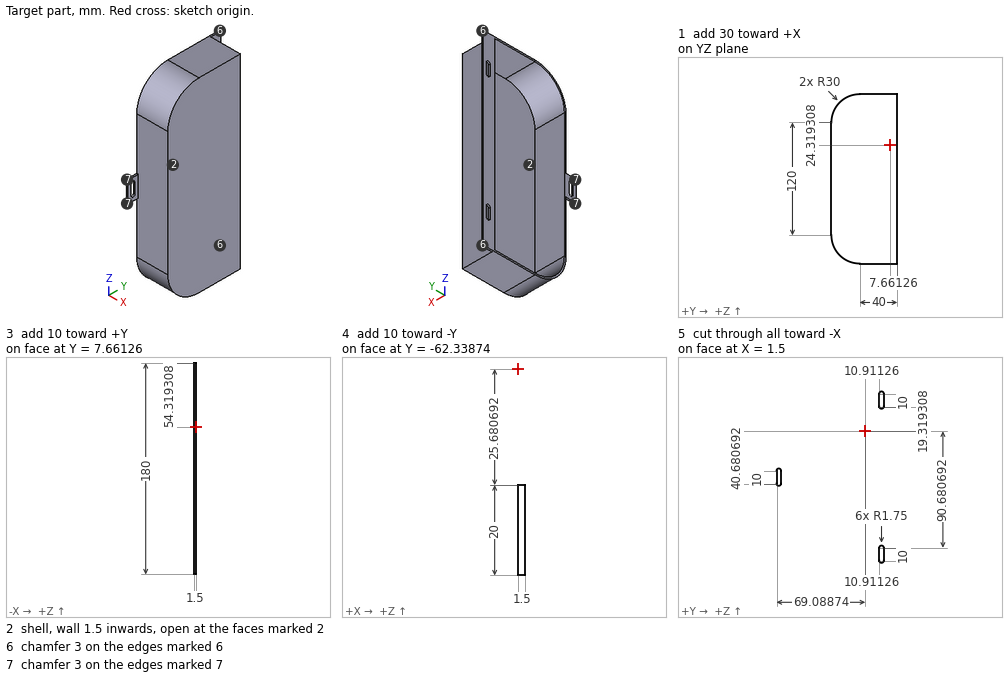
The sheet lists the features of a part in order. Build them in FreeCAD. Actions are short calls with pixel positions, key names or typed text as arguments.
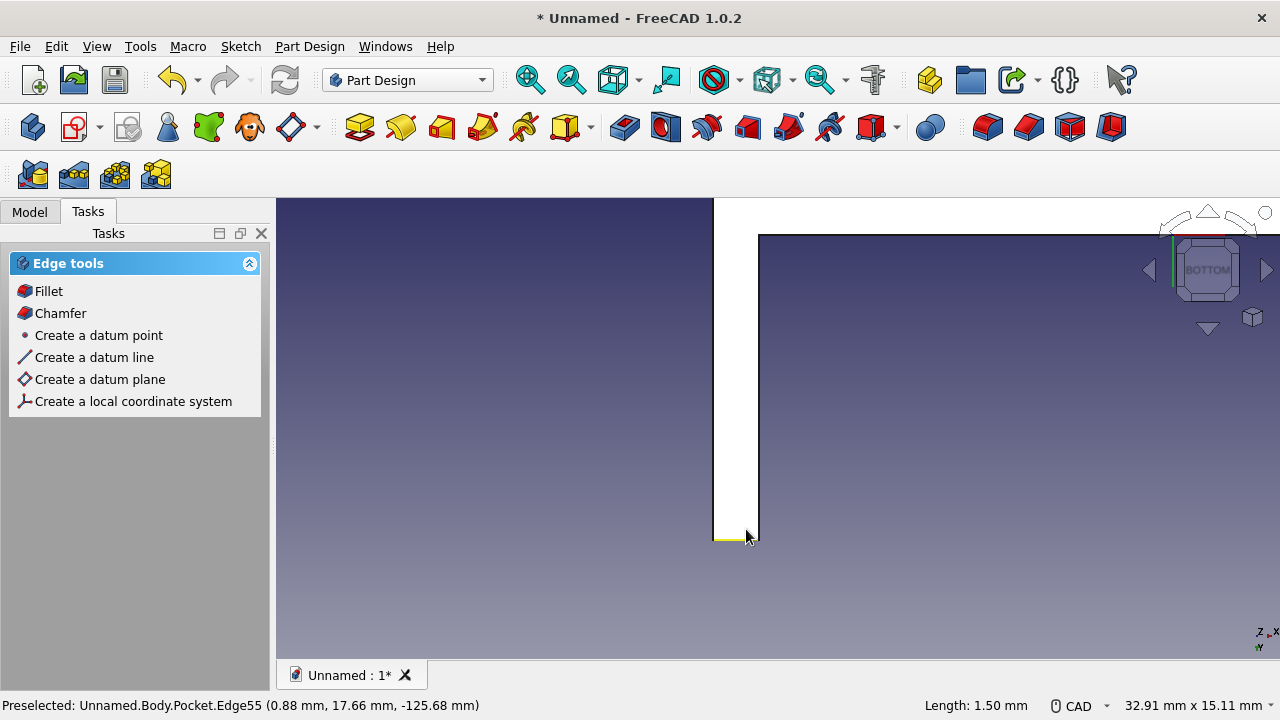
click(736, 539, ctrl)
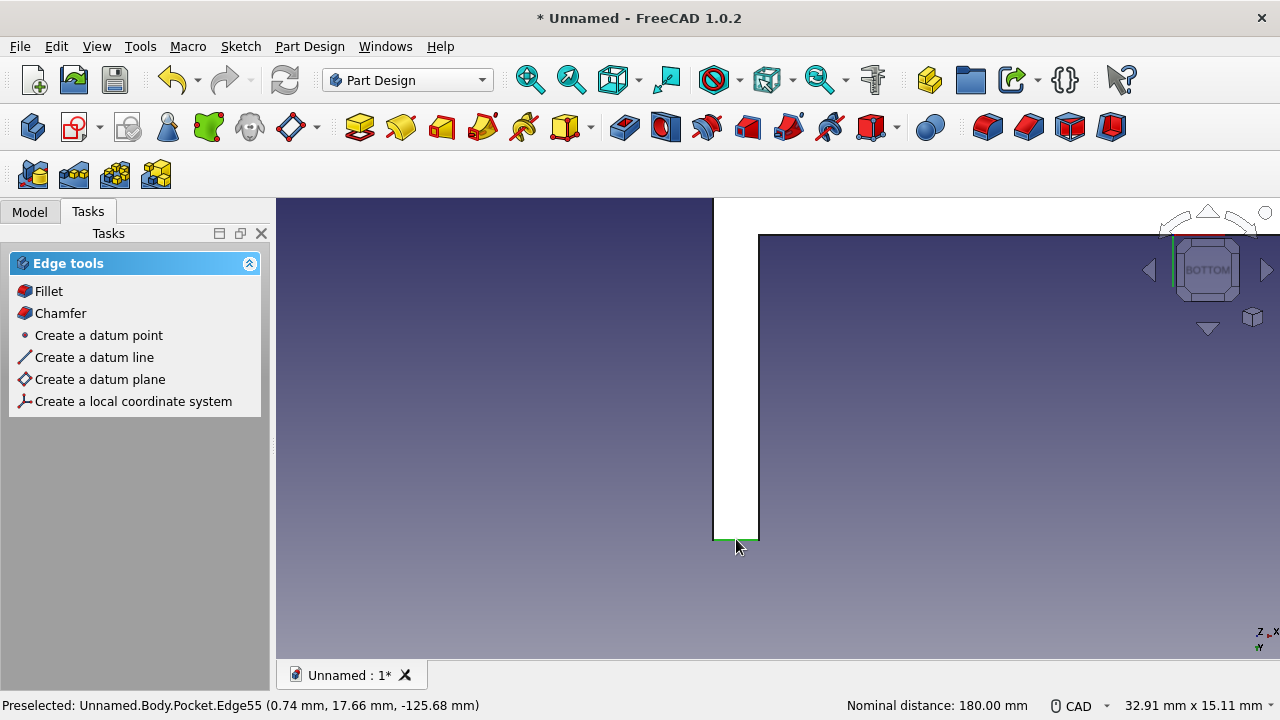
click(1029, 128)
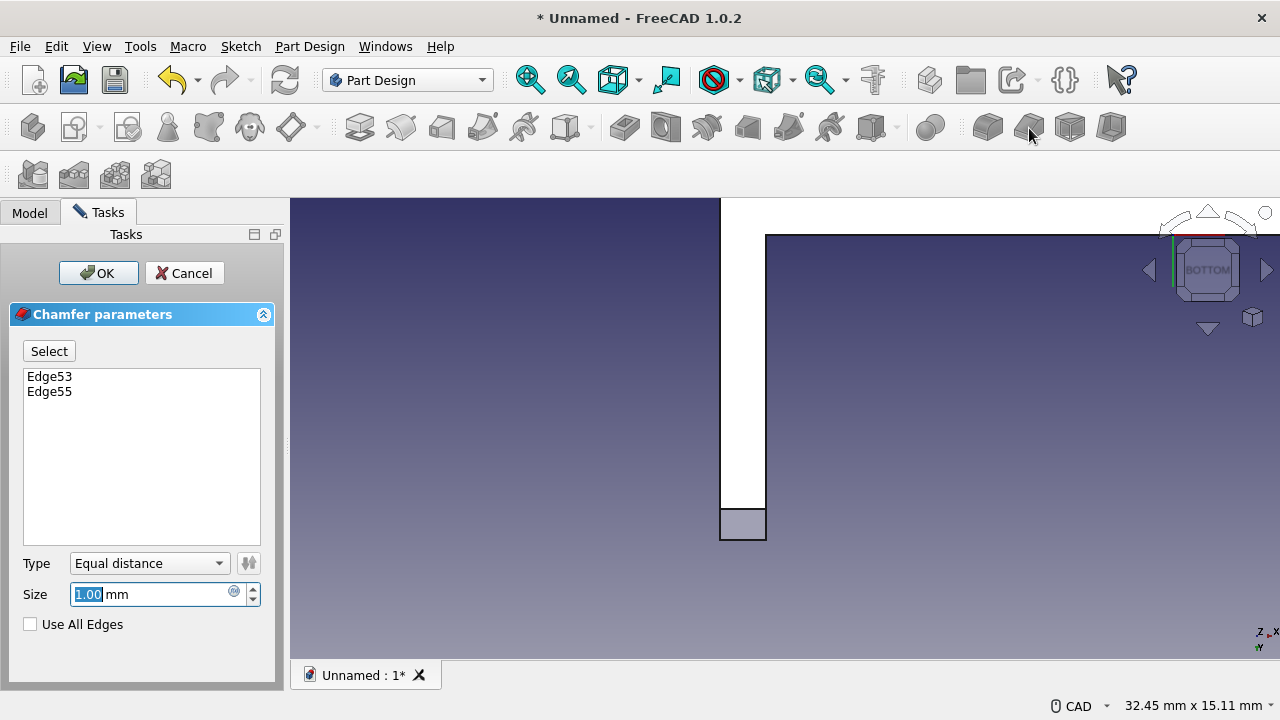
text(3)
key(Tab)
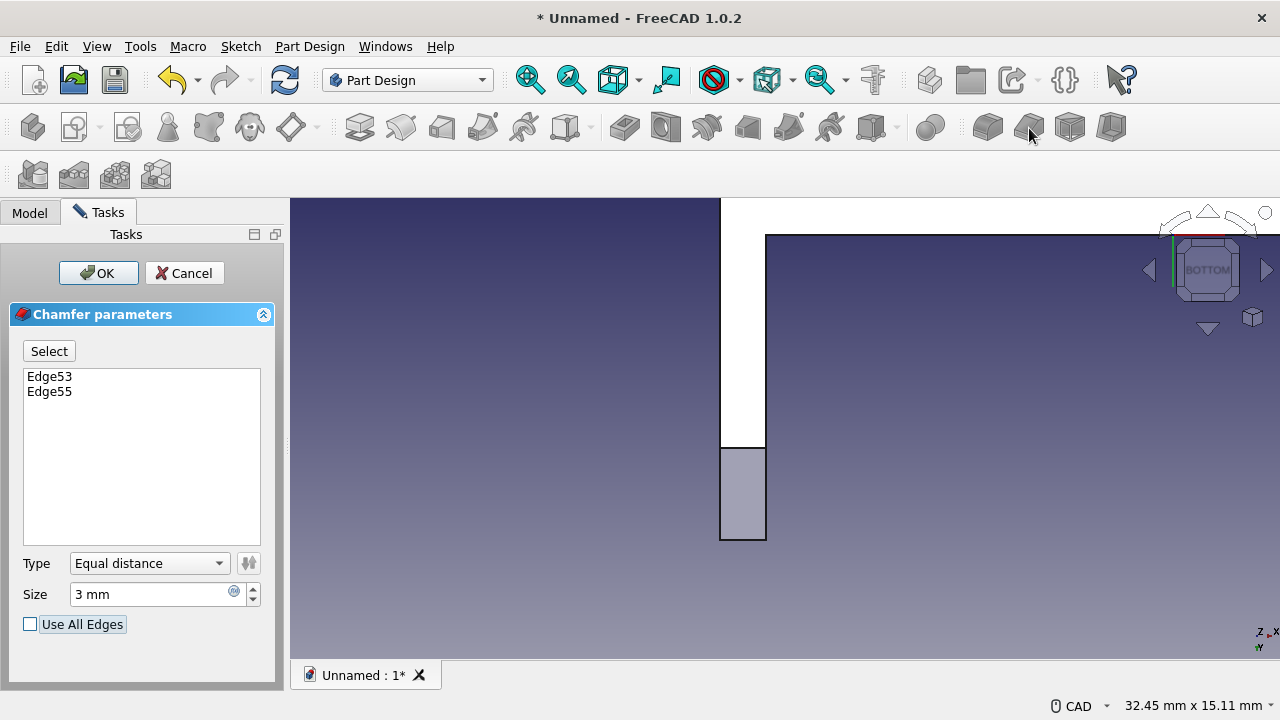
click(99, 273)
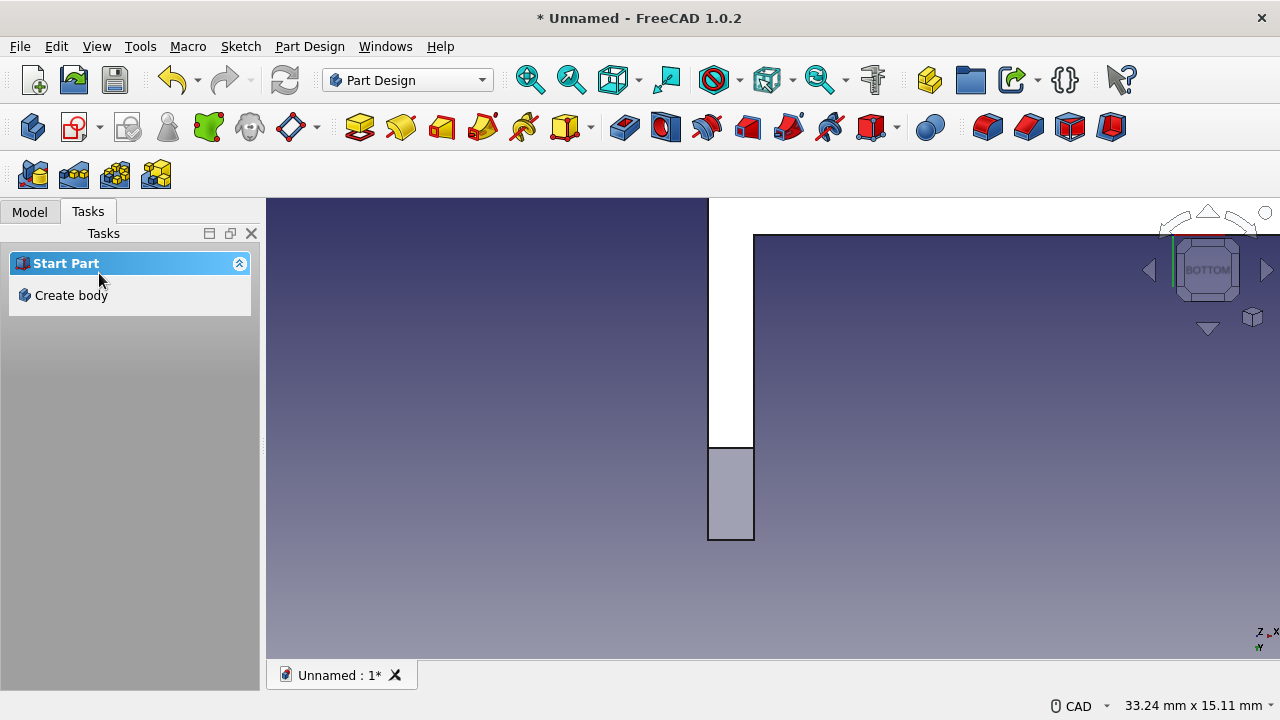
click(531, 80)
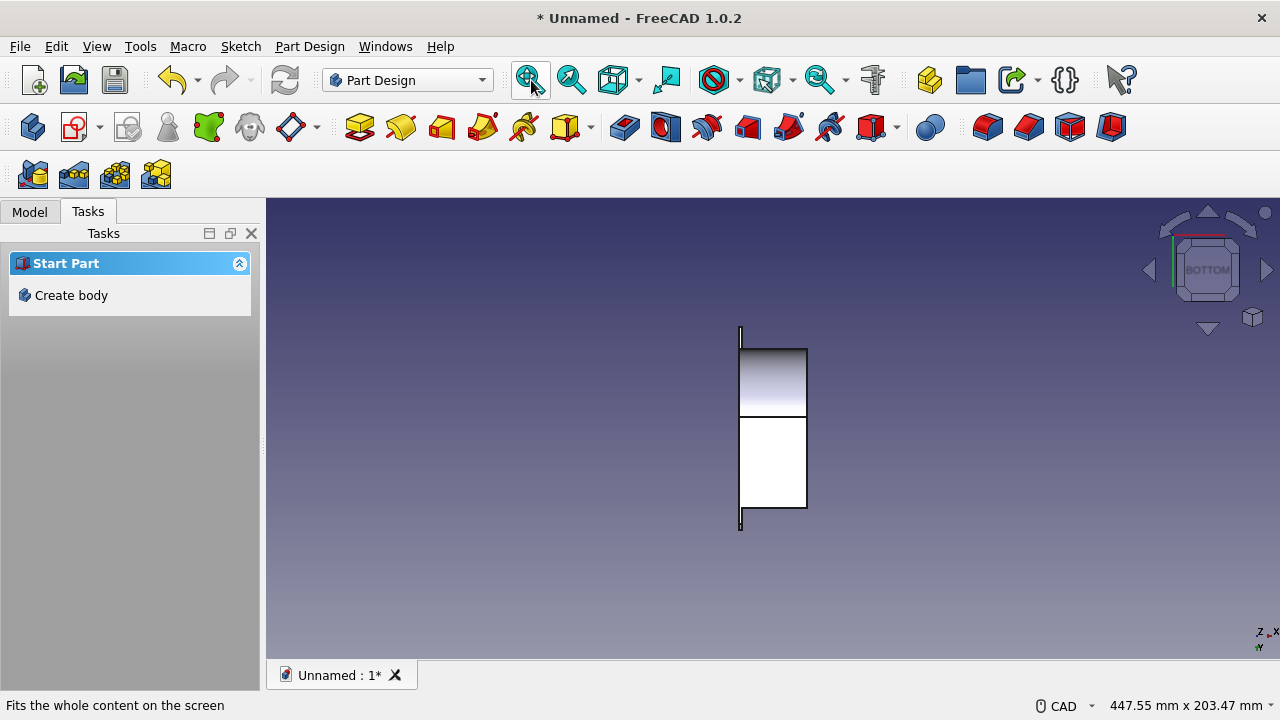
scroll(741, 326, up, 13)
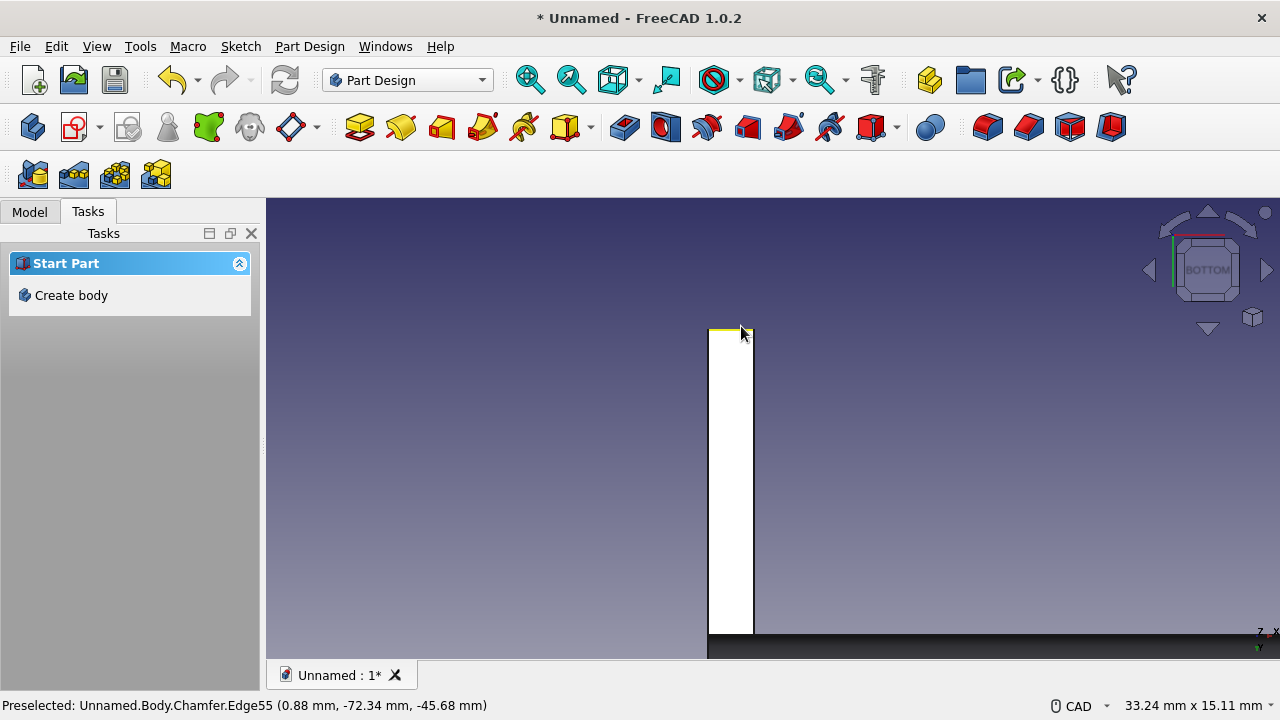
click(731, 329)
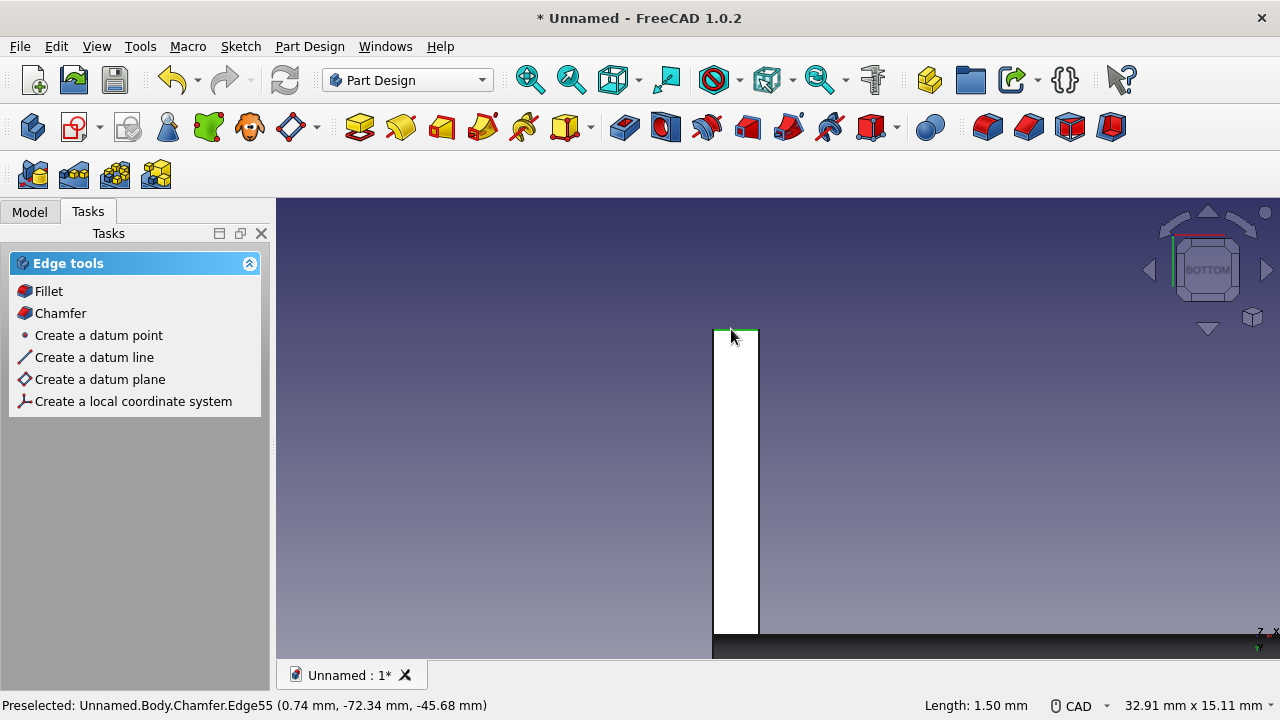
click(531, 80)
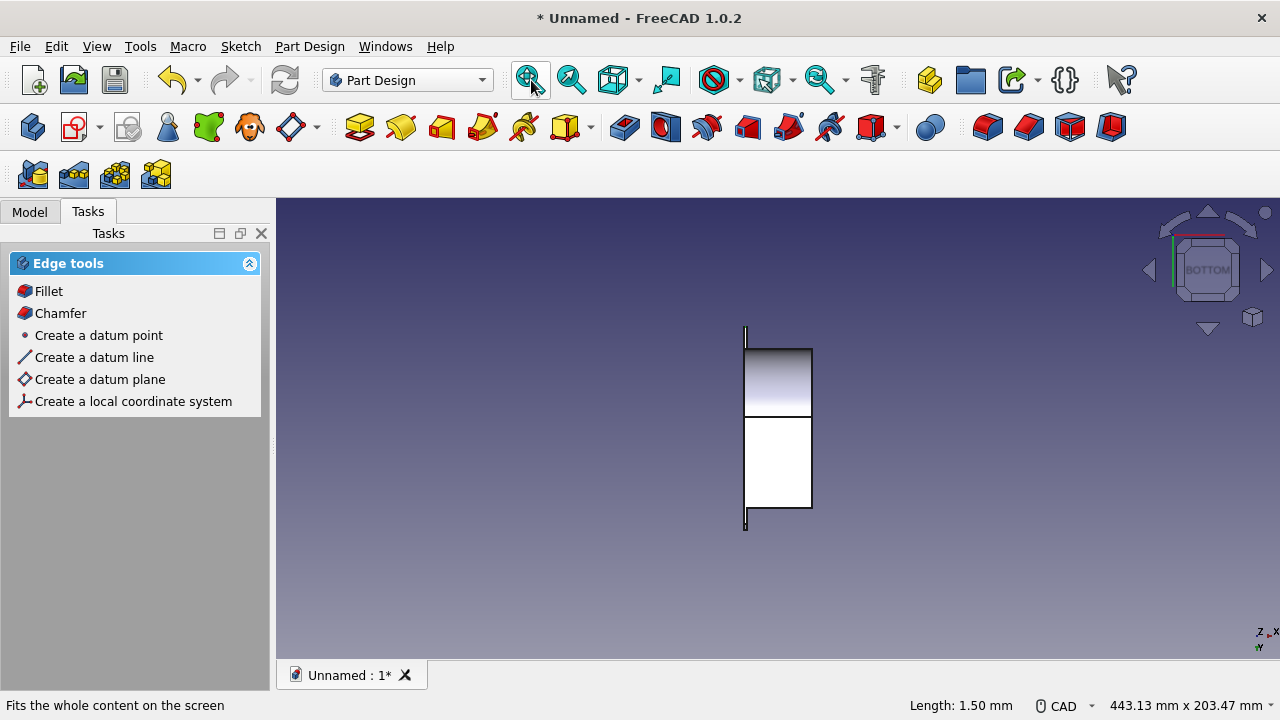
key(0)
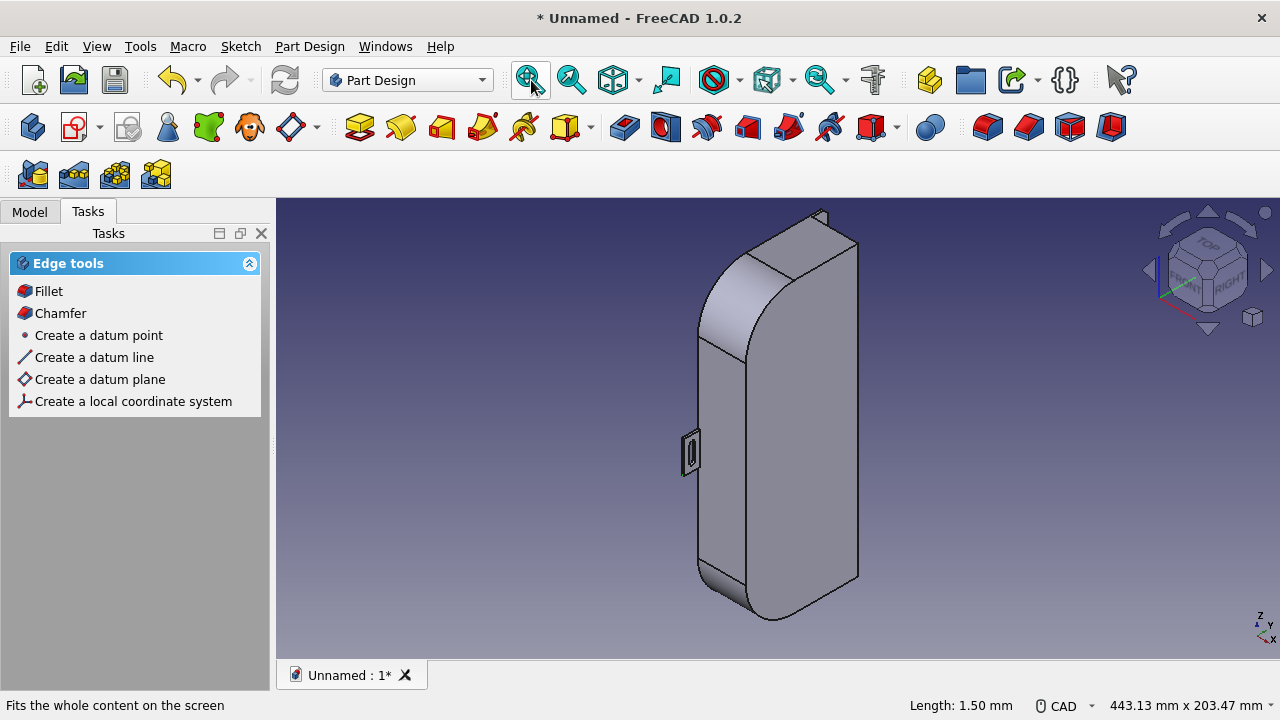
scroll(683, 437, up, 13)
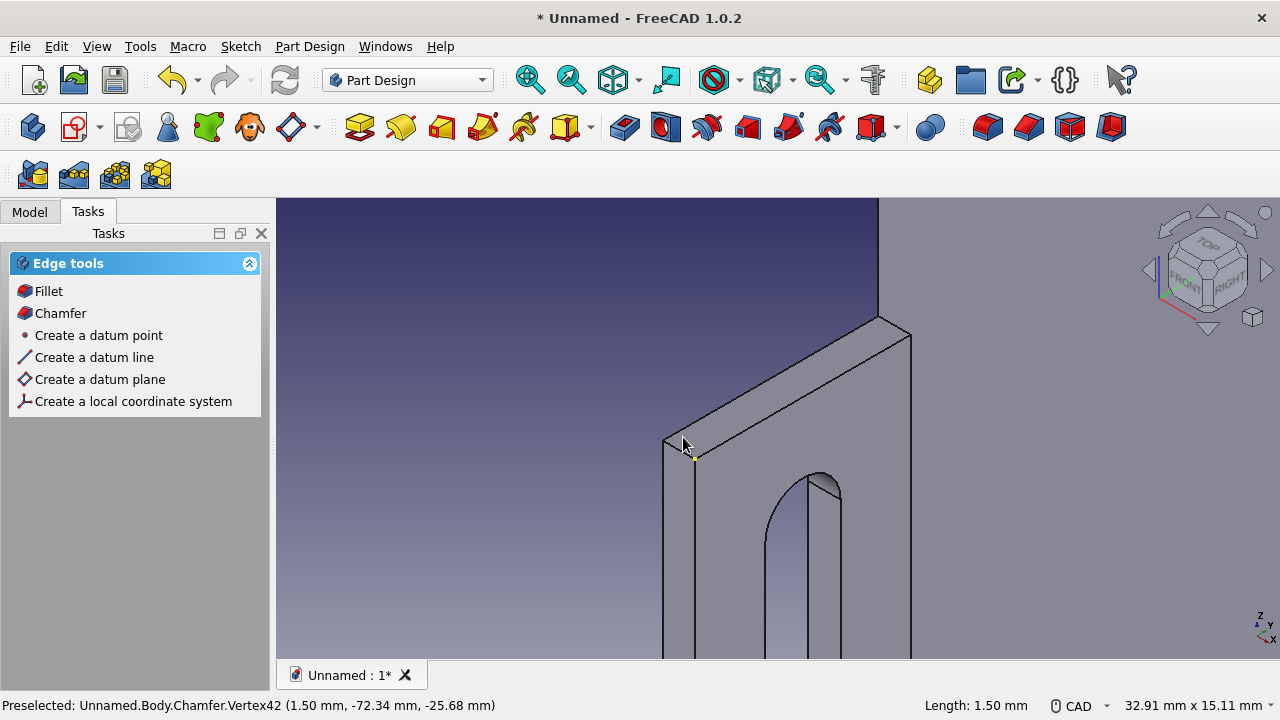
click(679, 449, ctrl)